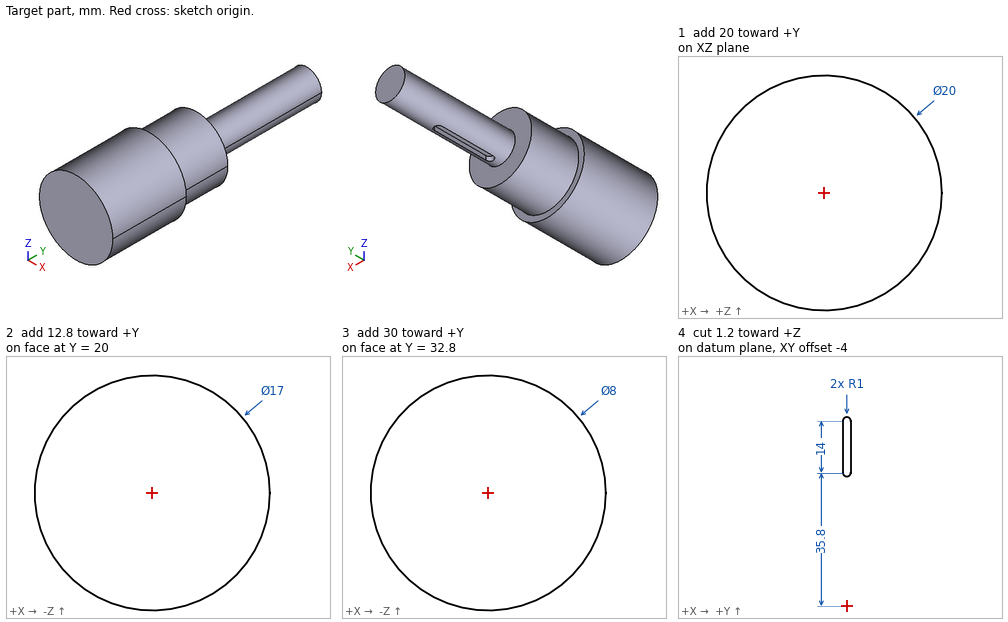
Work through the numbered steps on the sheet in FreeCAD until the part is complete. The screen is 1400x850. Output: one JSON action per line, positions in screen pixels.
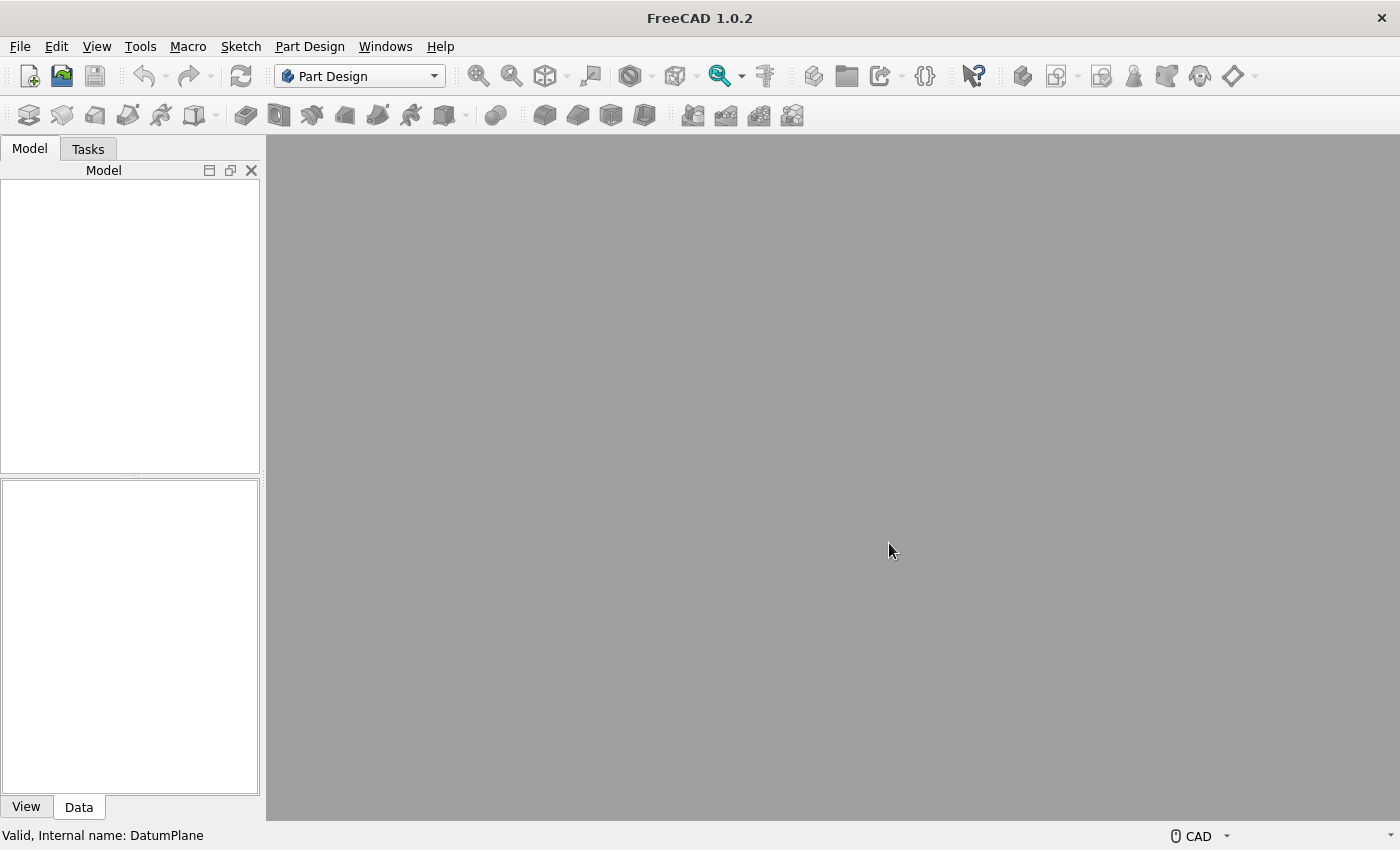
{"action": "left_click", "coordinate": [29, 76]}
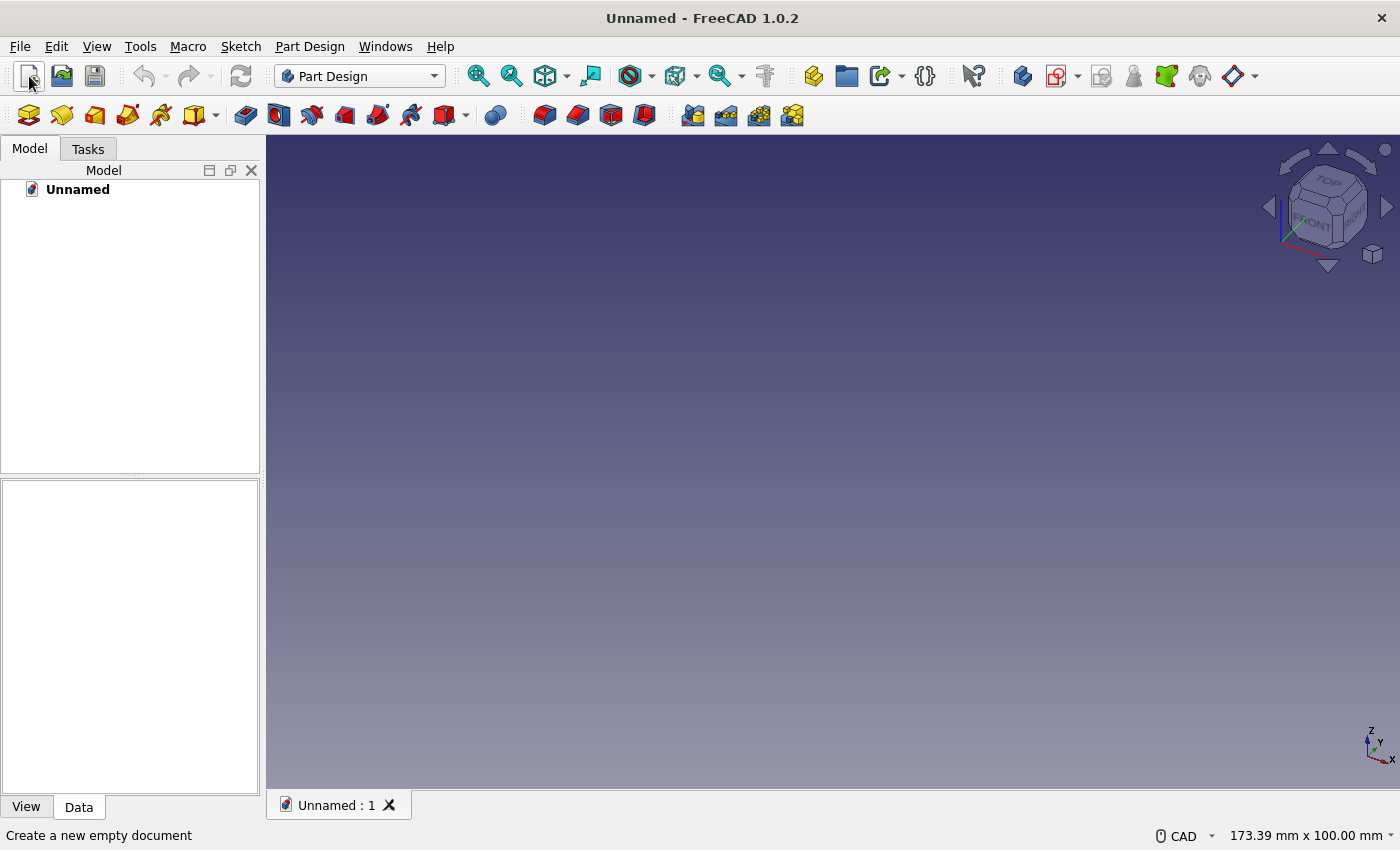
{"action": "left_click", "coordinate": [1056, 76]}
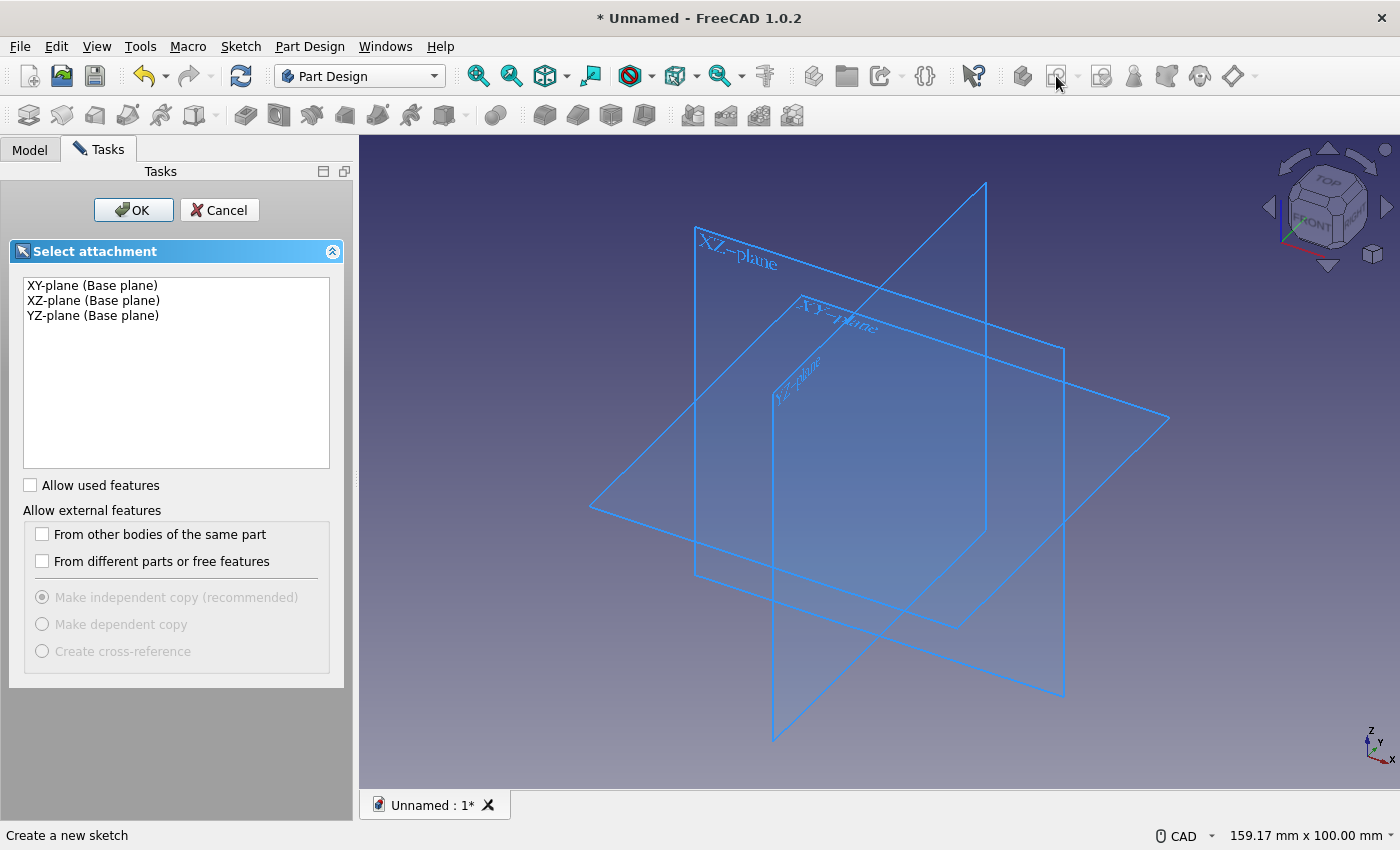
{"action": "left_click", "coordinate": [84, 300]}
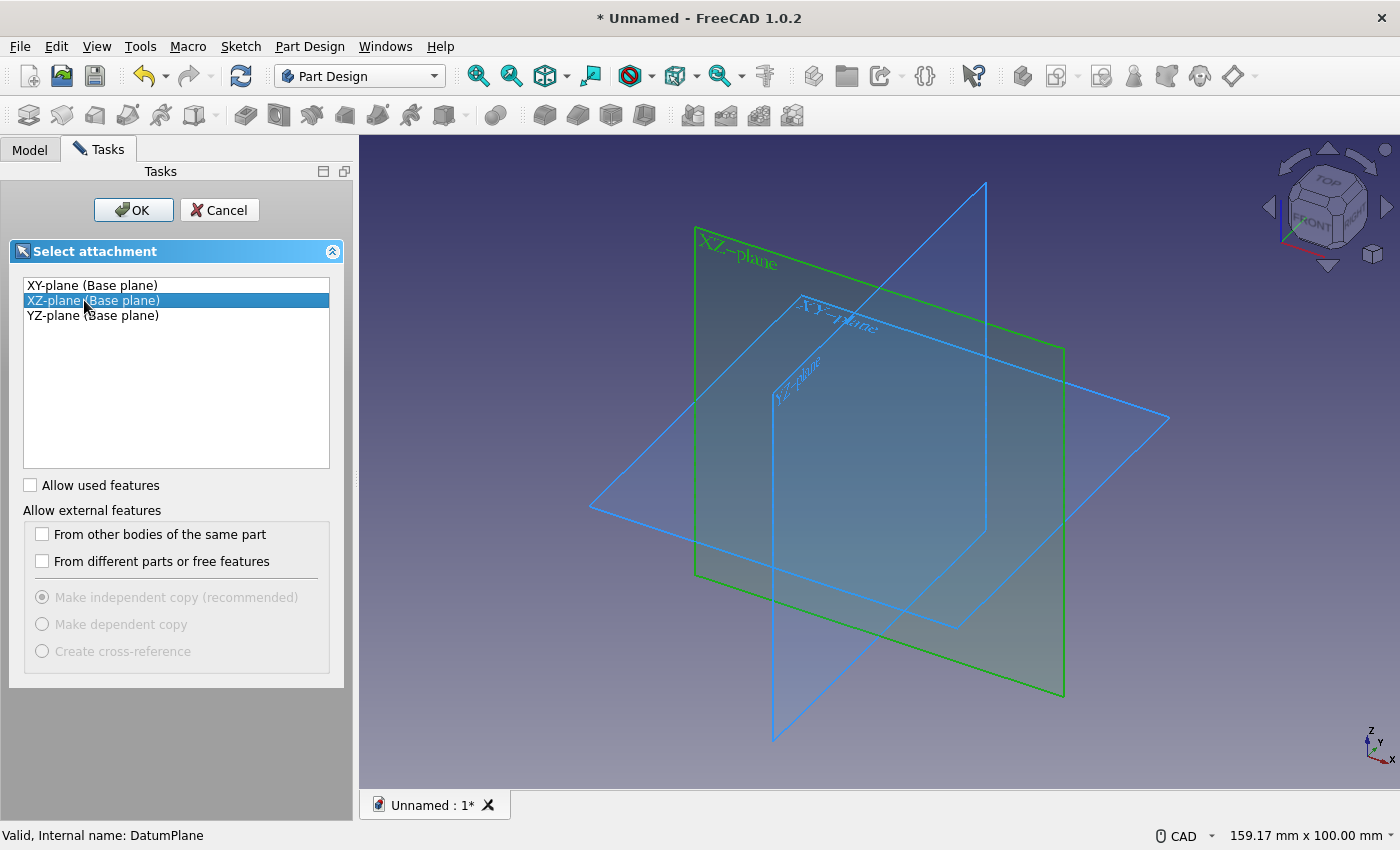
{"action": "left_click", "coordinate": [134, 210]}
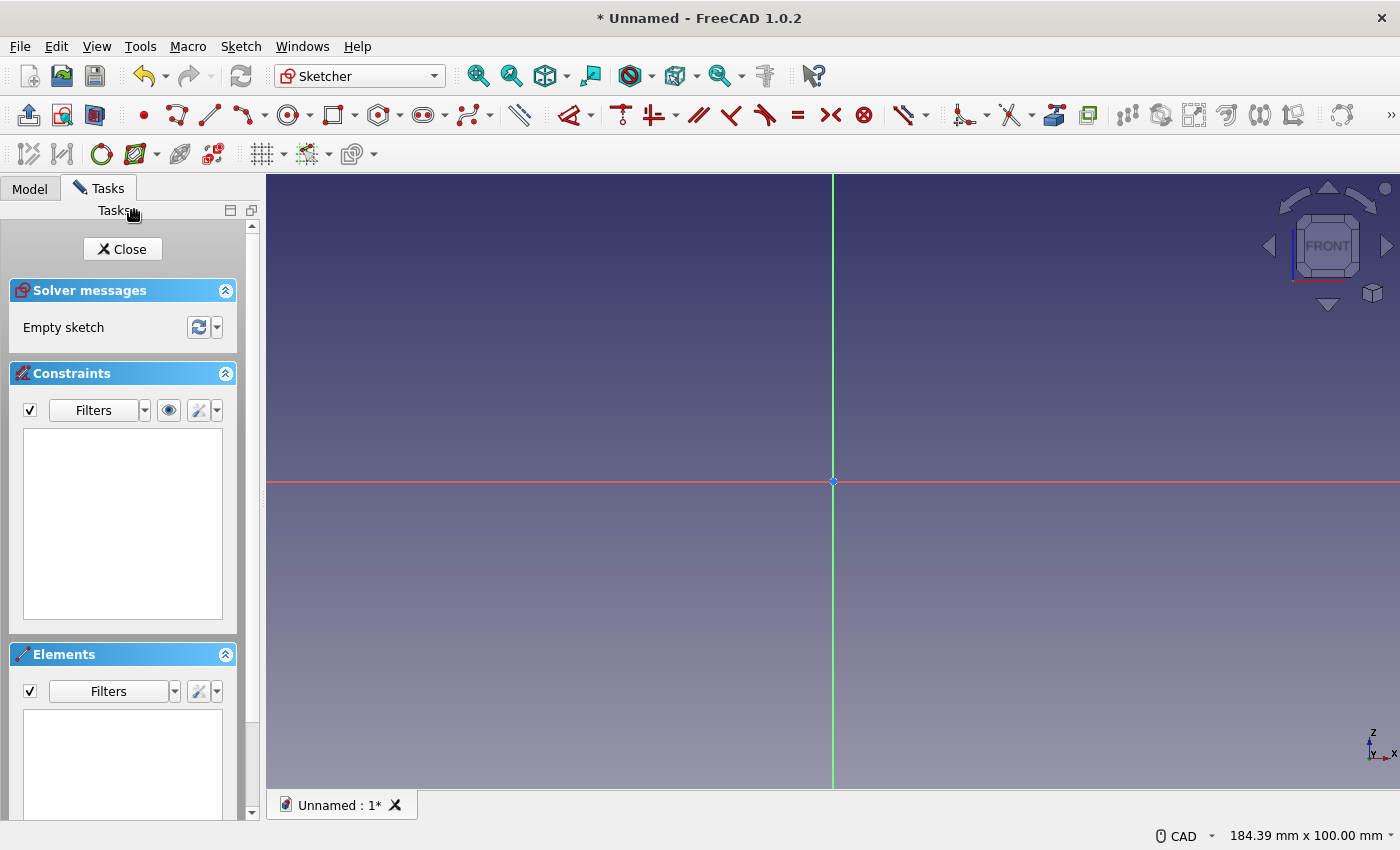
{"action": "scroll", "coordinate": [863, 482], "scroll_direction": "up", "scroll_amount": 6}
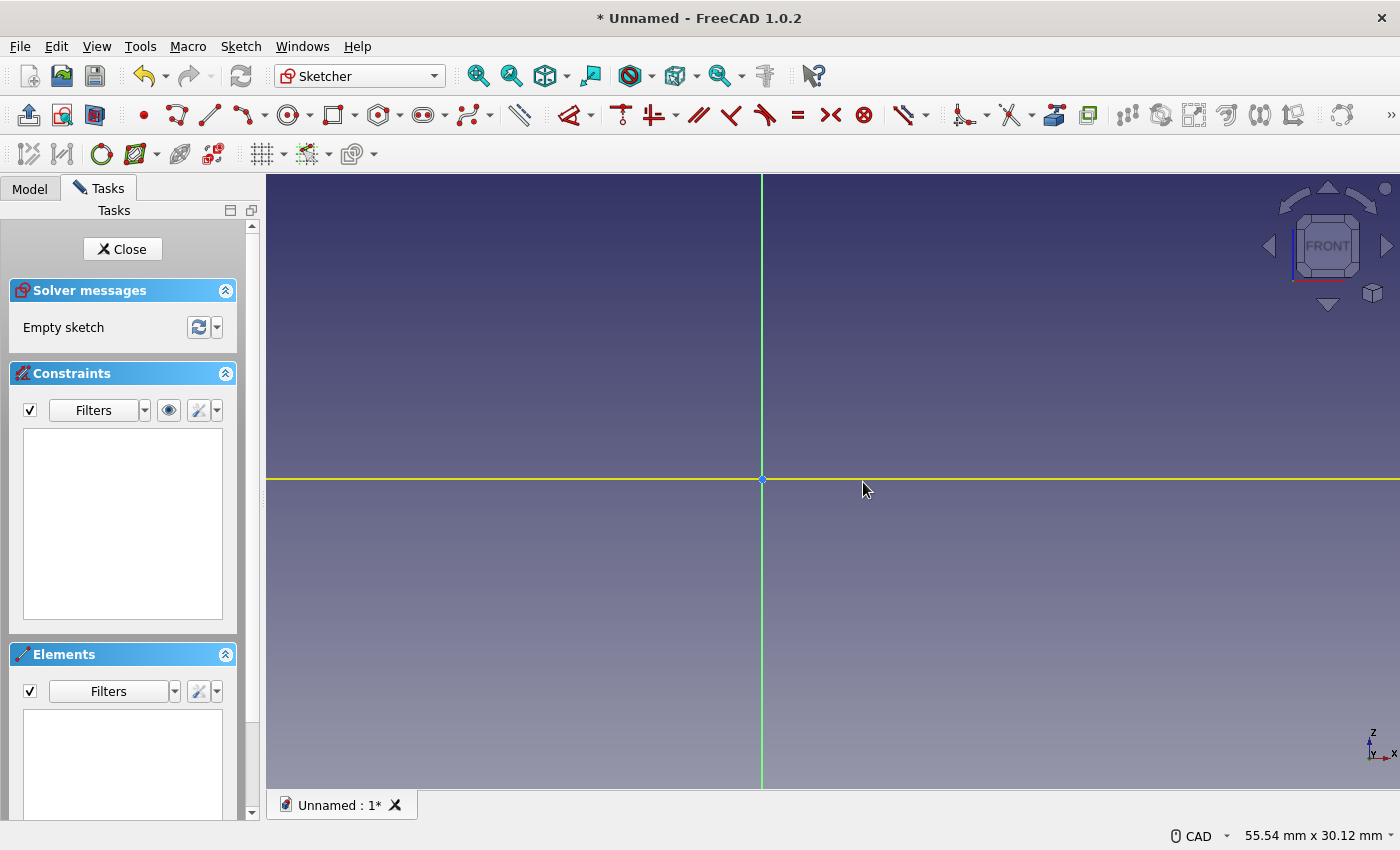
{"action": "left_click", "coordinate": [288, 116]}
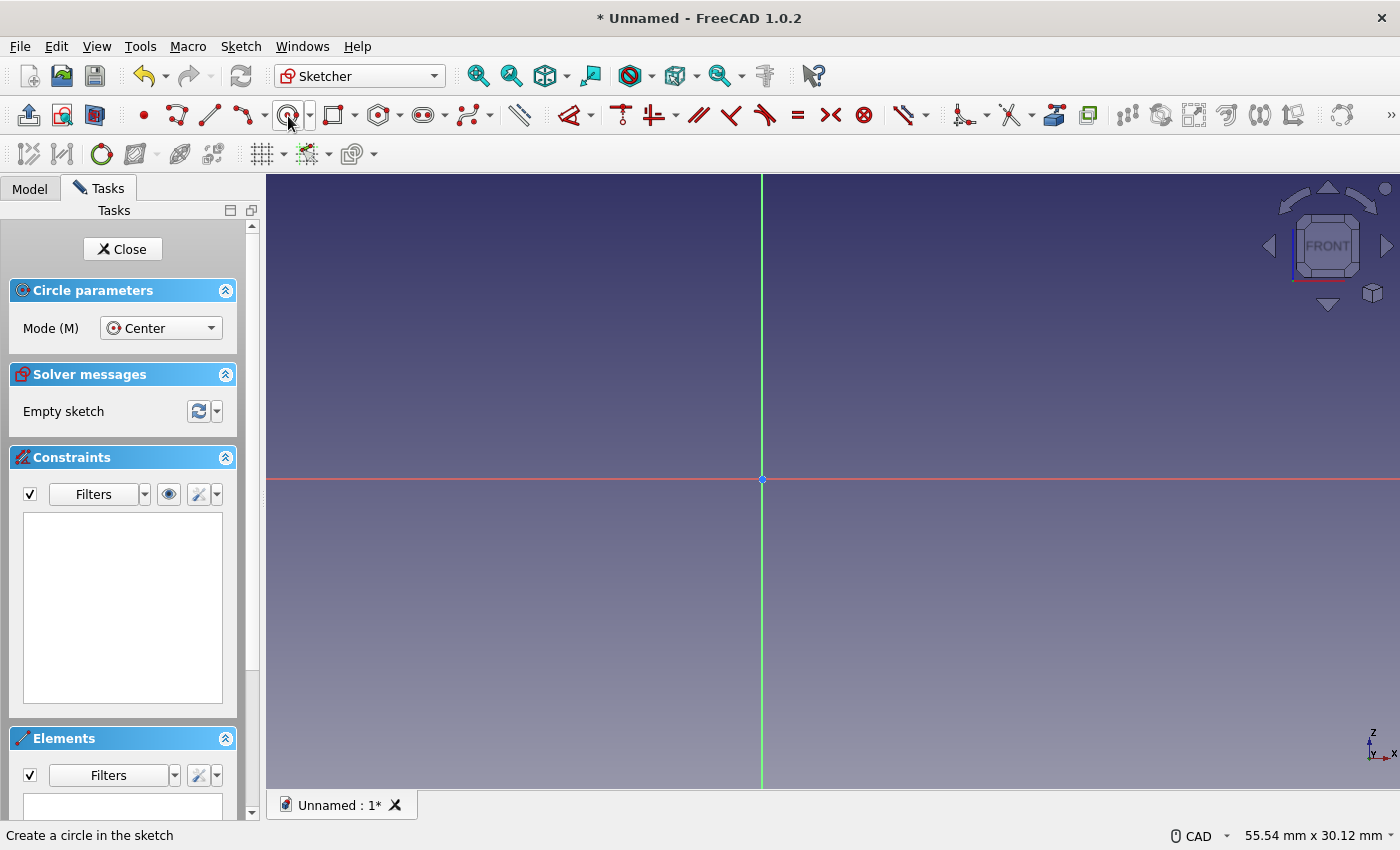
{"action": "left_click", "coordinate": [762, 479]}
{"action": "mouse_move", "coordinate": [907, 335]}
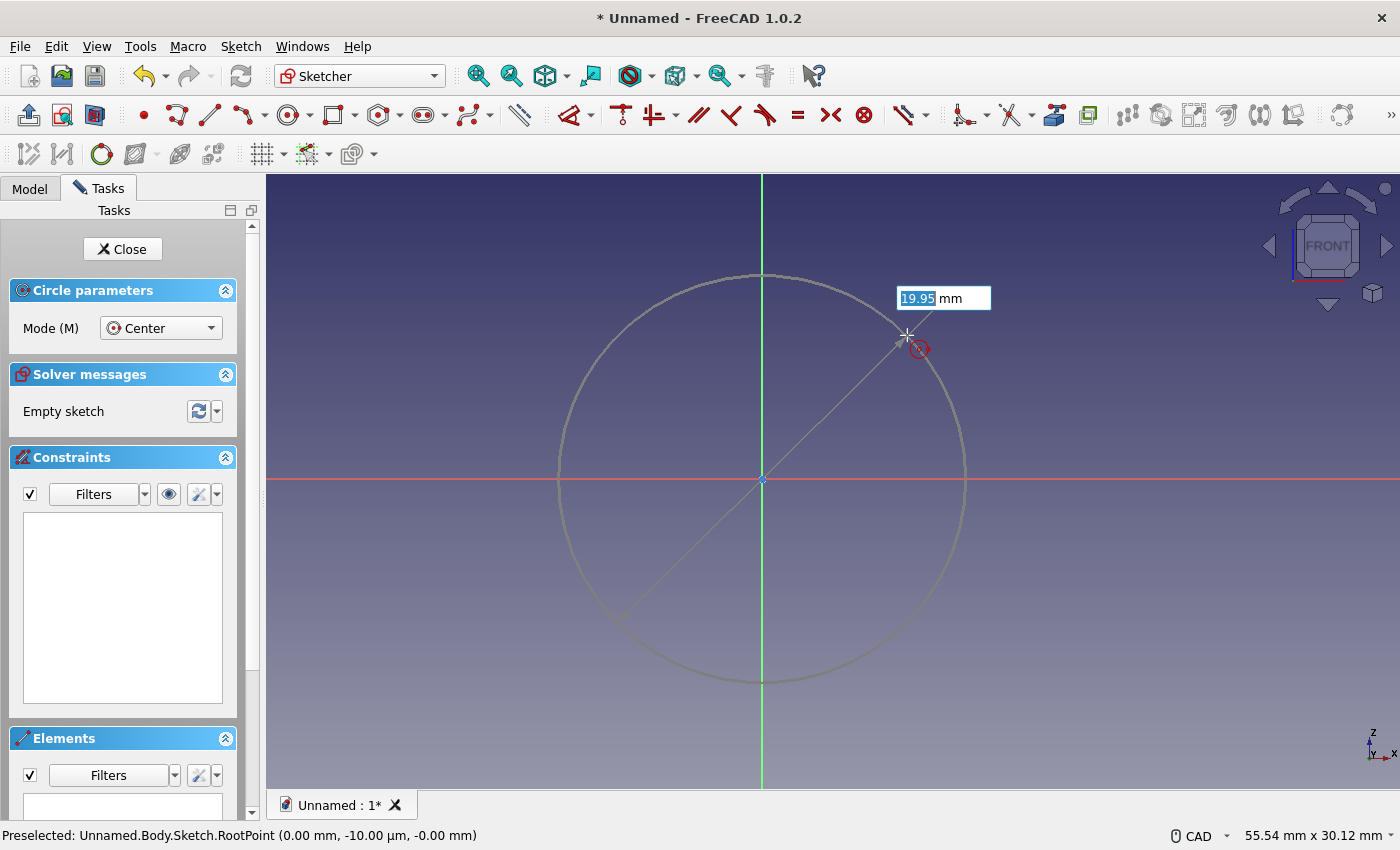
{"action": "type", "text": "20"}
{"action": "key", "text": "Return"}
{"action": "key", "text": "Escape"}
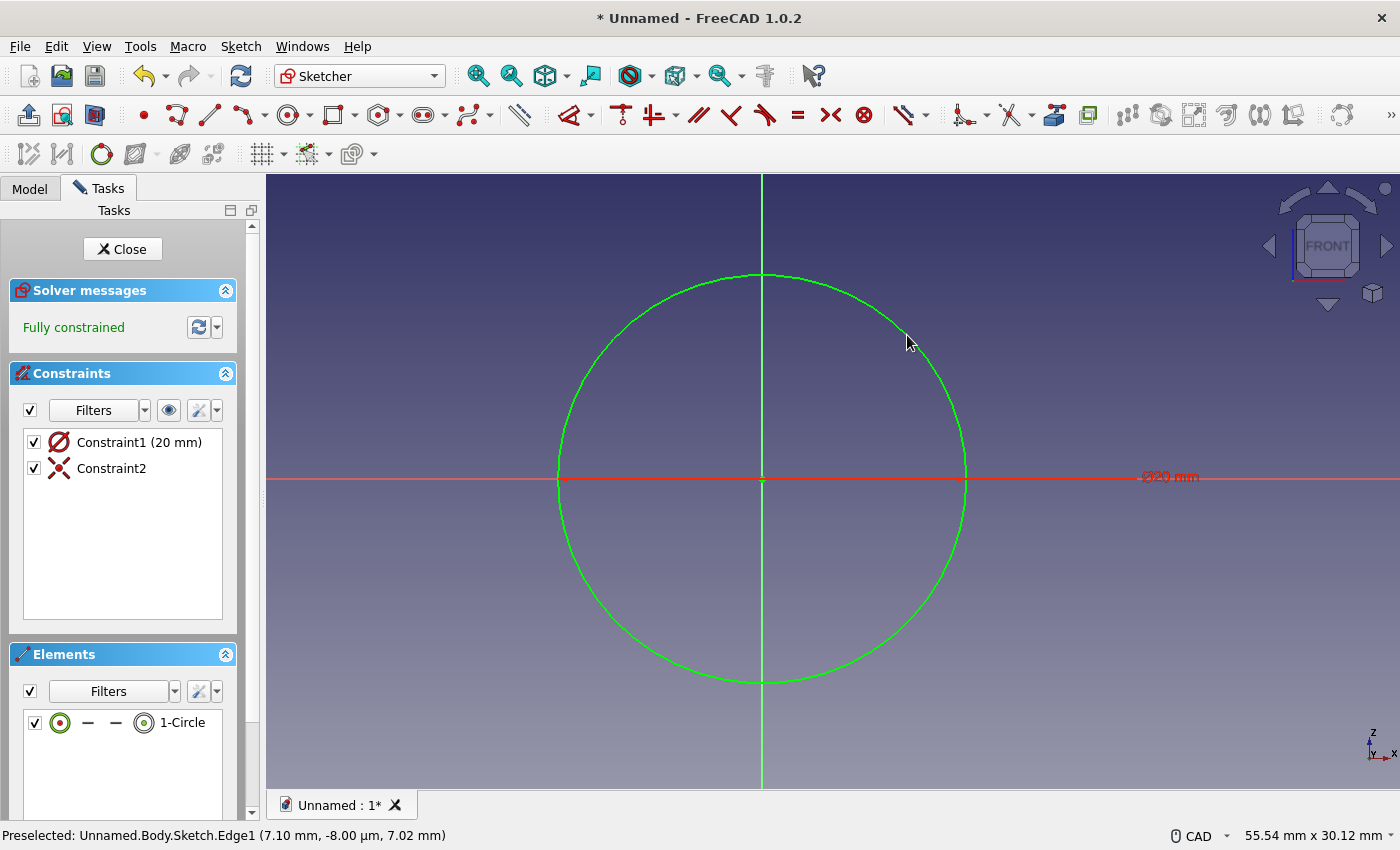
{"action": "left_click", "coordinate": [123, 249]}